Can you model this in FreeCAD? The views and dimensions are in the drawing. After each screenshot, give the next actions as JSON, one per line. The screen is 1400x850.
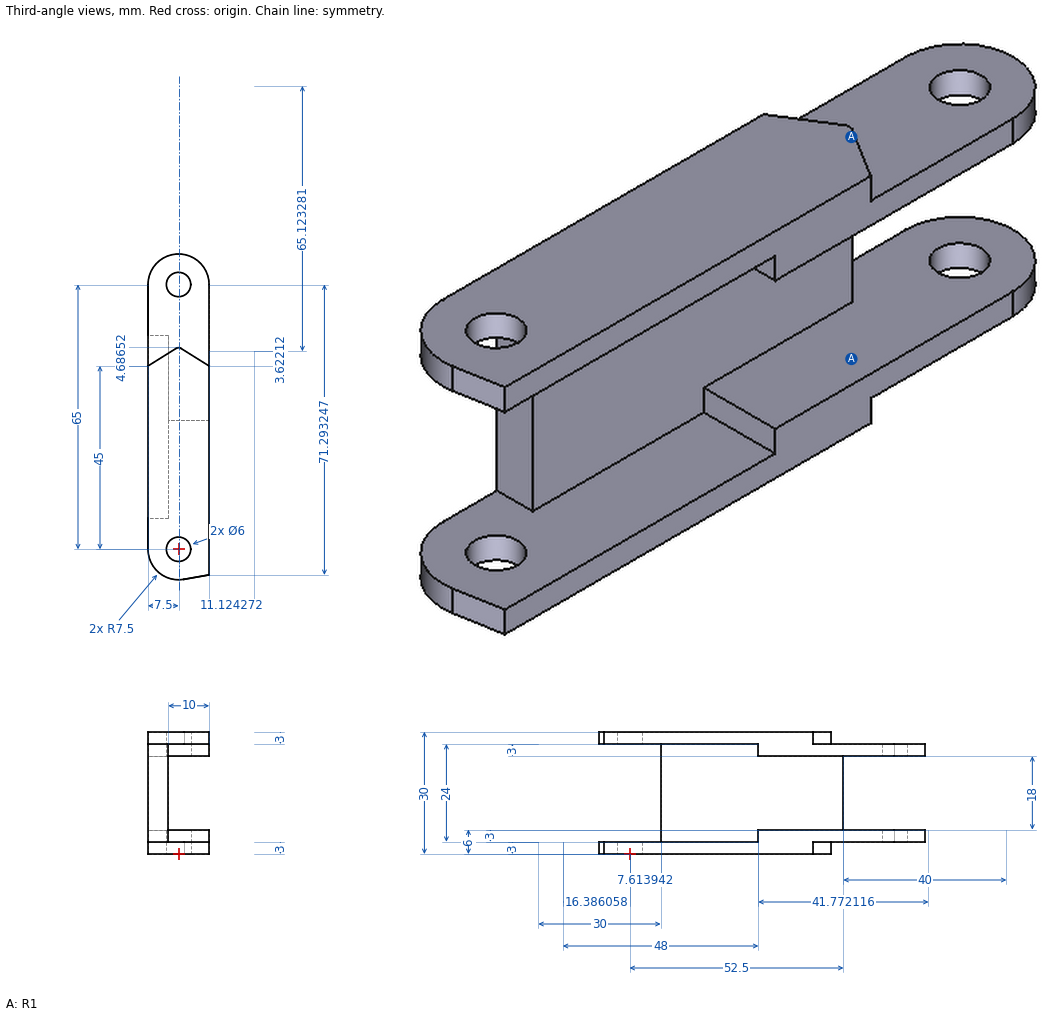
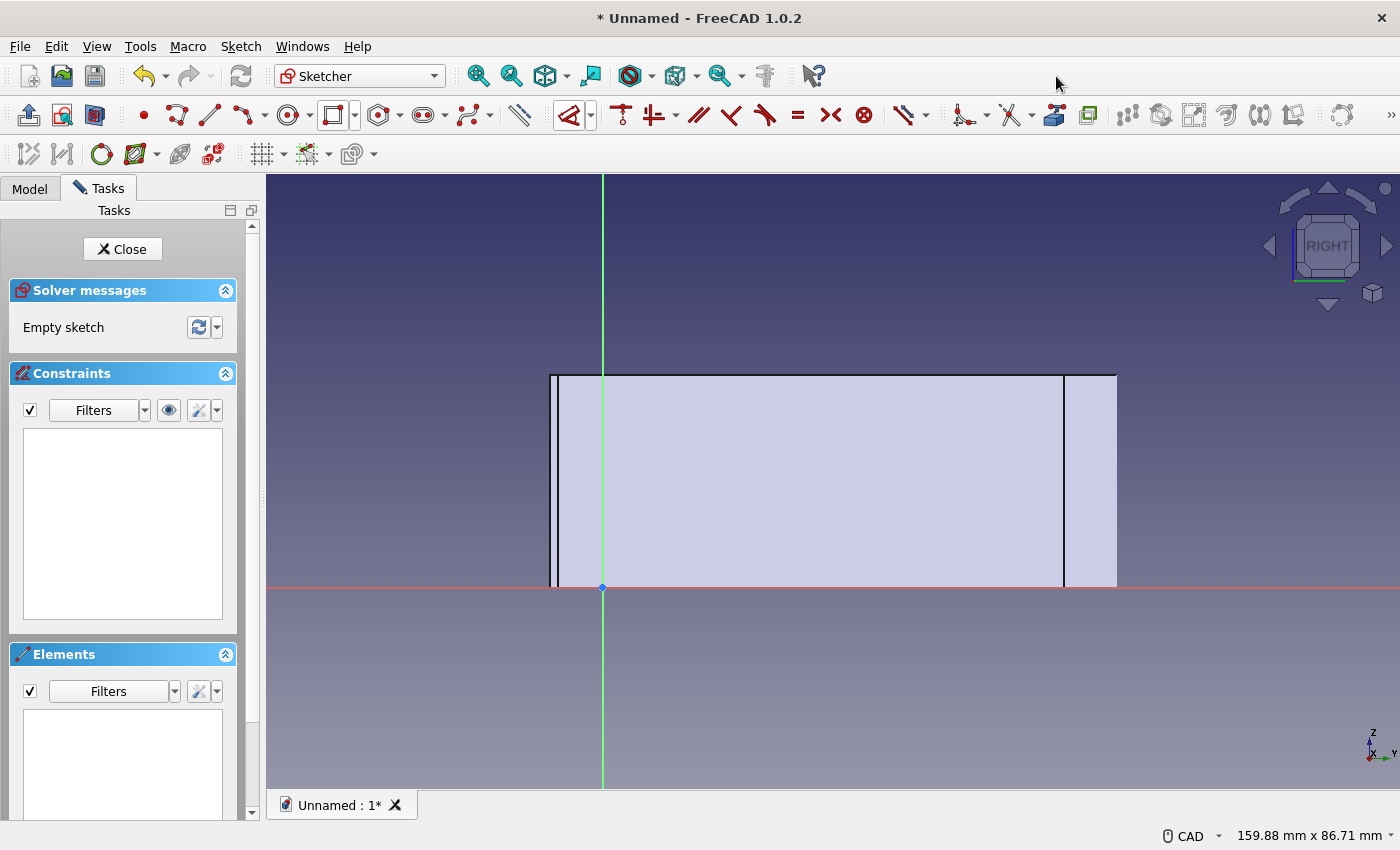
{"action": "scroll", "coordinate": [373, 433], "scroll_direction": "down", "scroll_amount": 1}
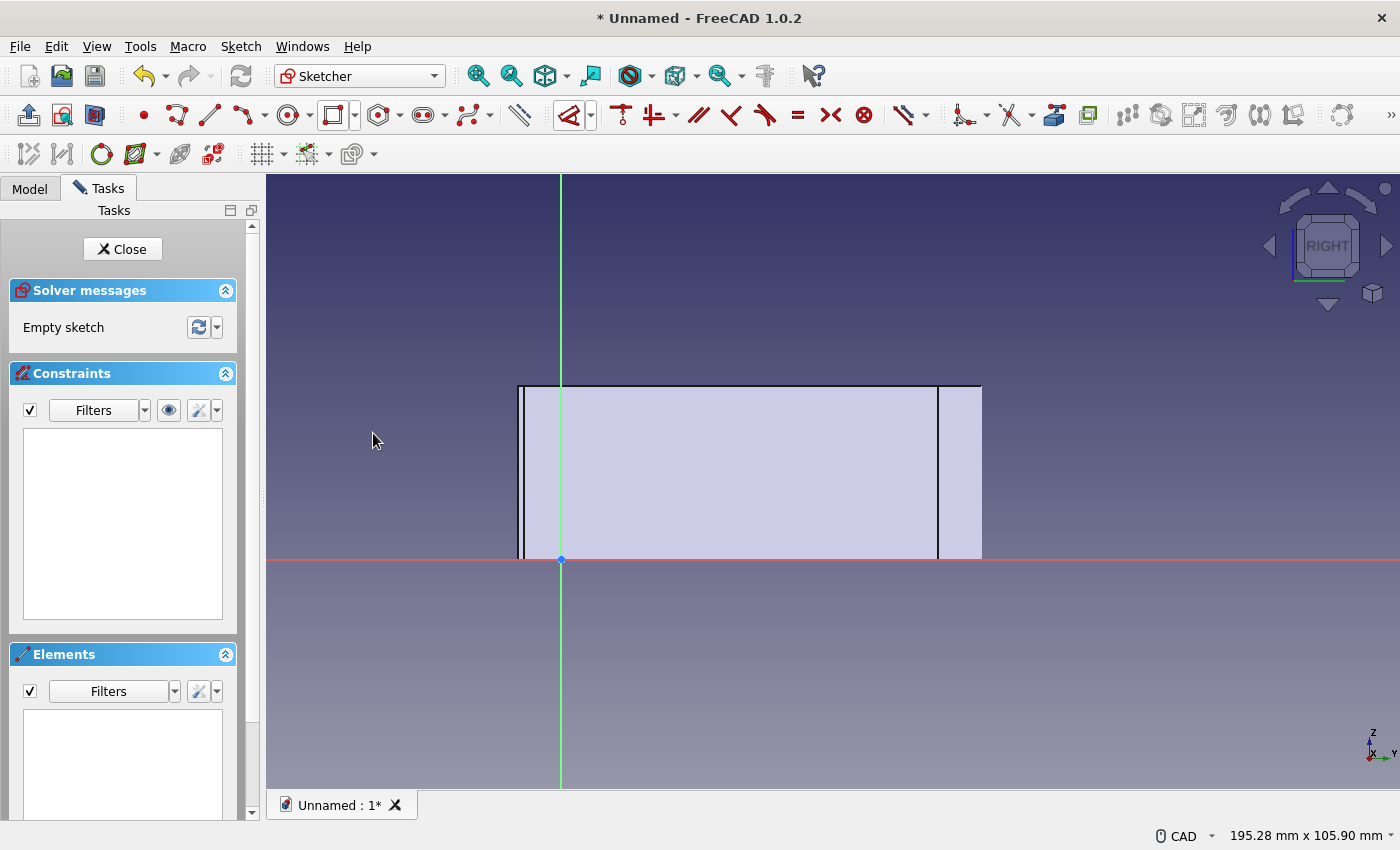
{"action": "key", "text": "g r"}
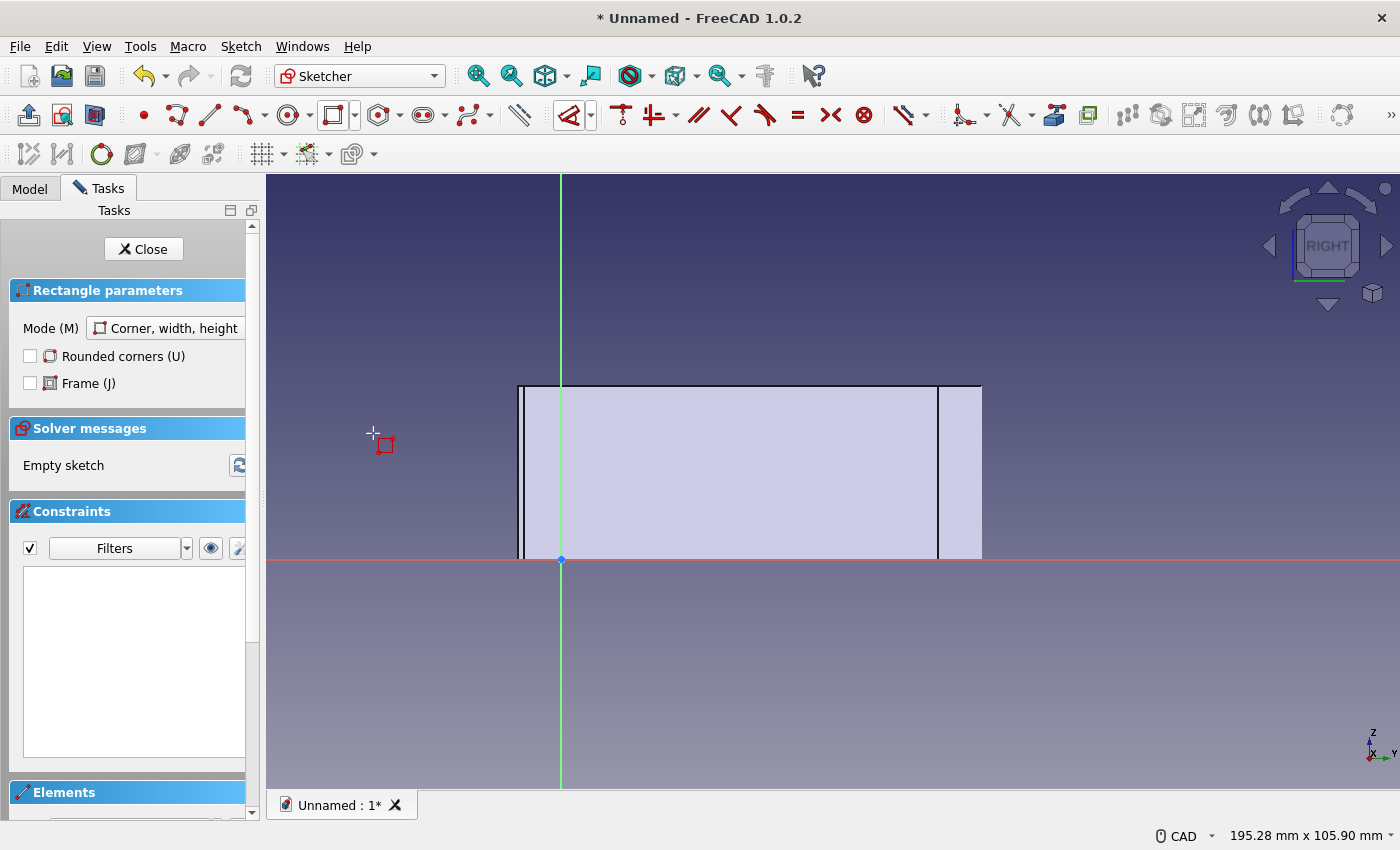
{"action": "left_click", "coordinate": [431, 403]}
{"action": "left_click", "coordinate": [605, 542]}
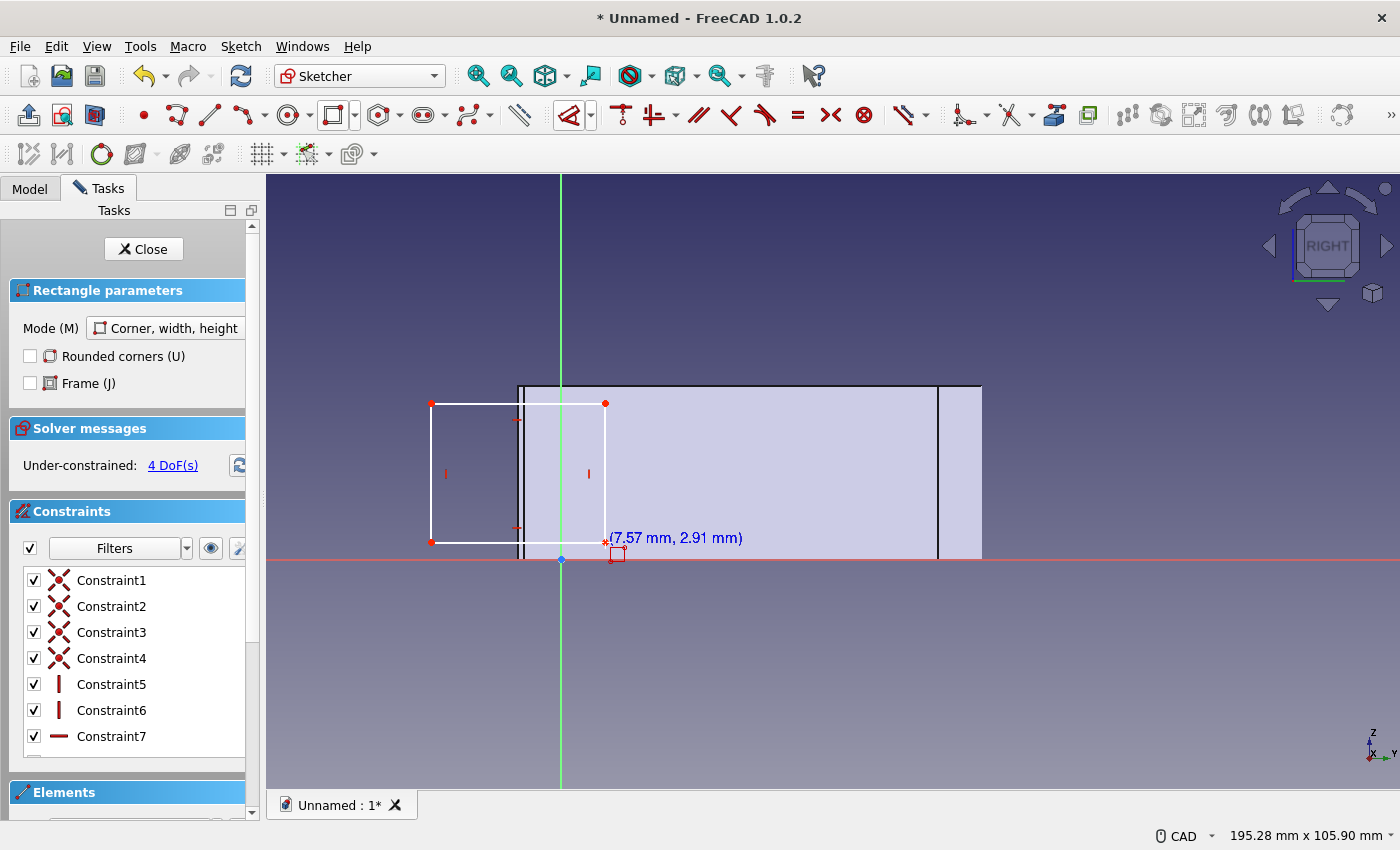
{"action": "left_click", "coordinate": [866, 421]}
{"action": "left_click", "coordinate": [1098, 525]}
{"action": "key", "text": "Escape"}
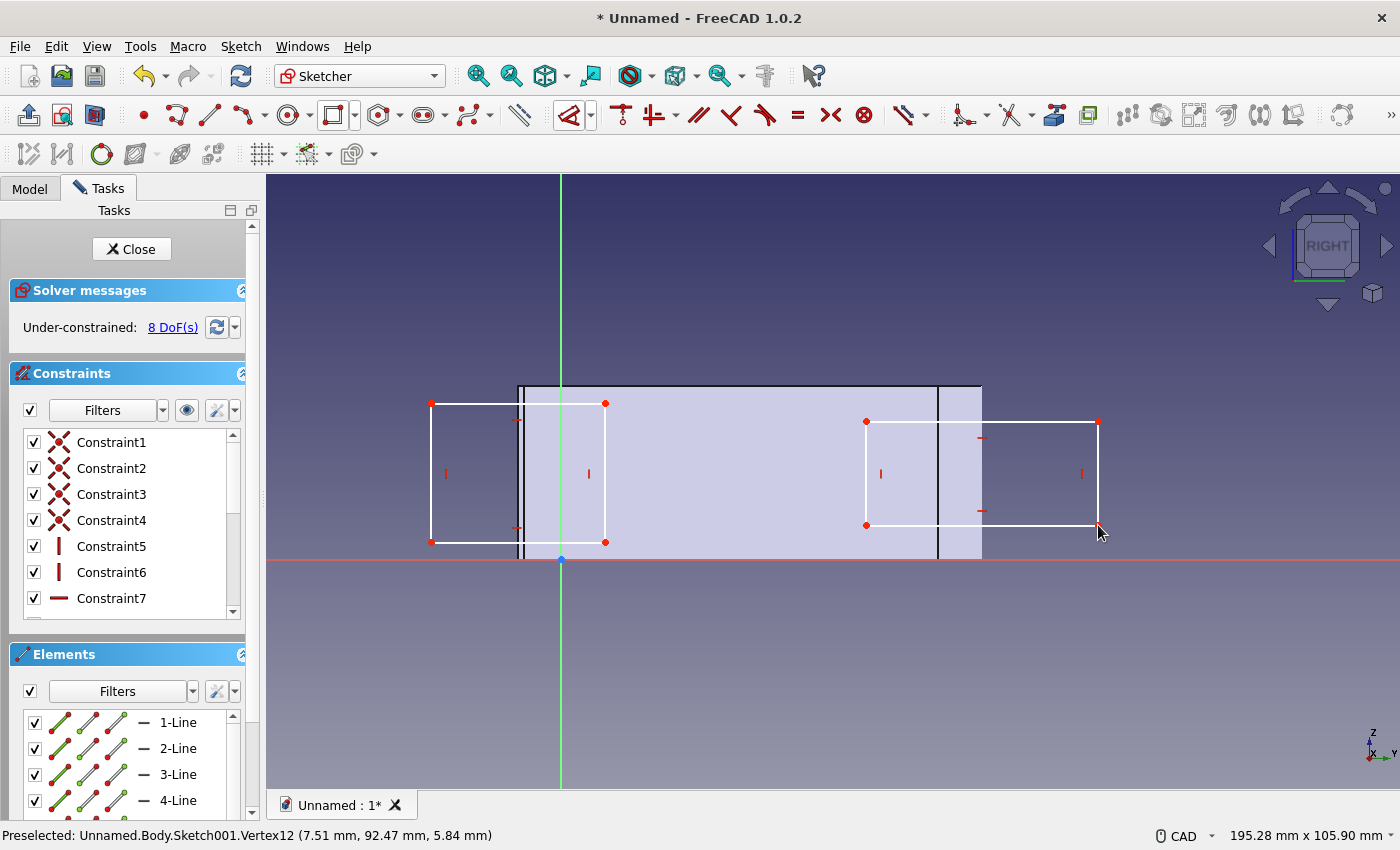
{"action": "left_click", "coordinate": [431, 446]}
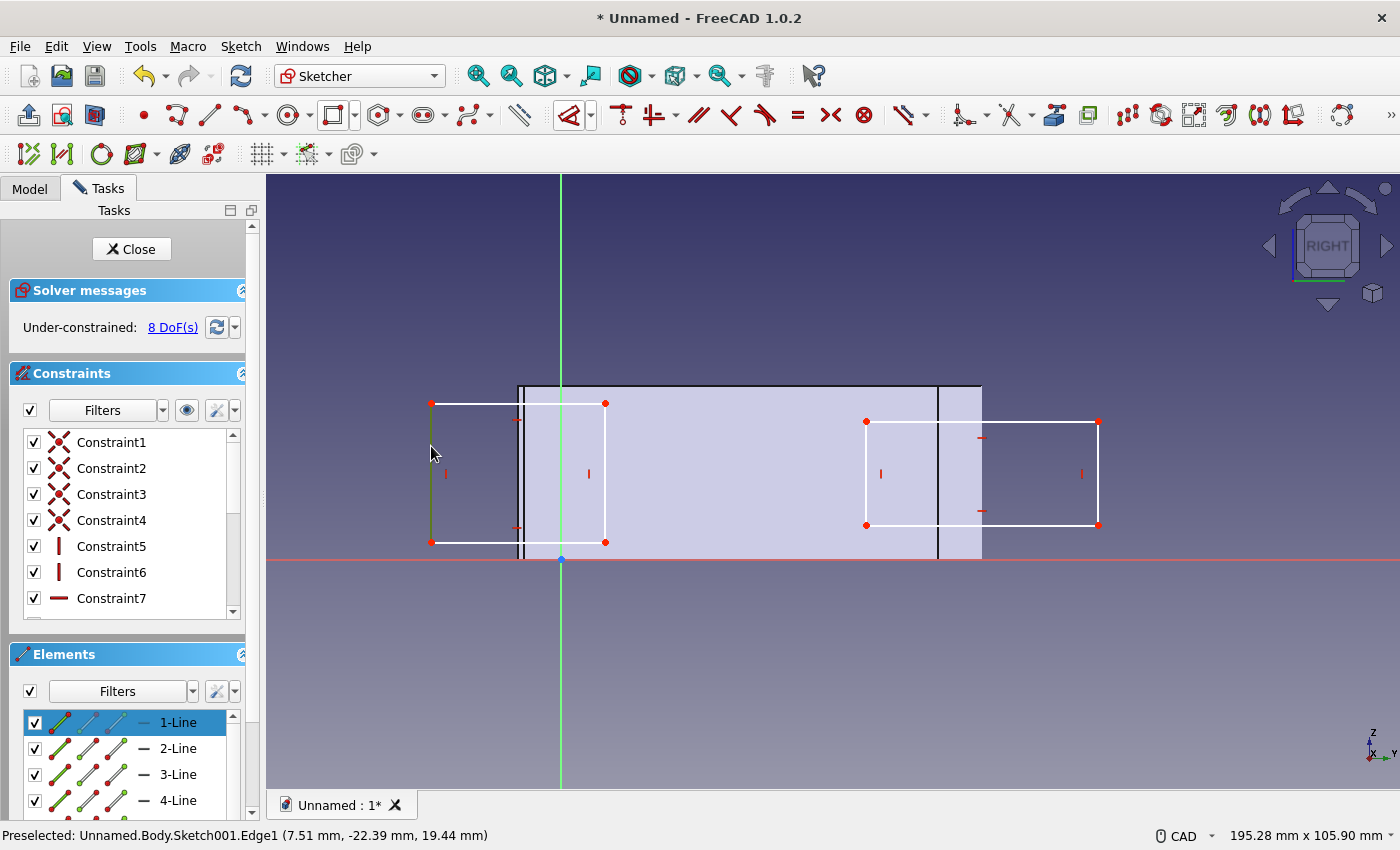
{"action": "left_click", "coordinate": [590, 116]}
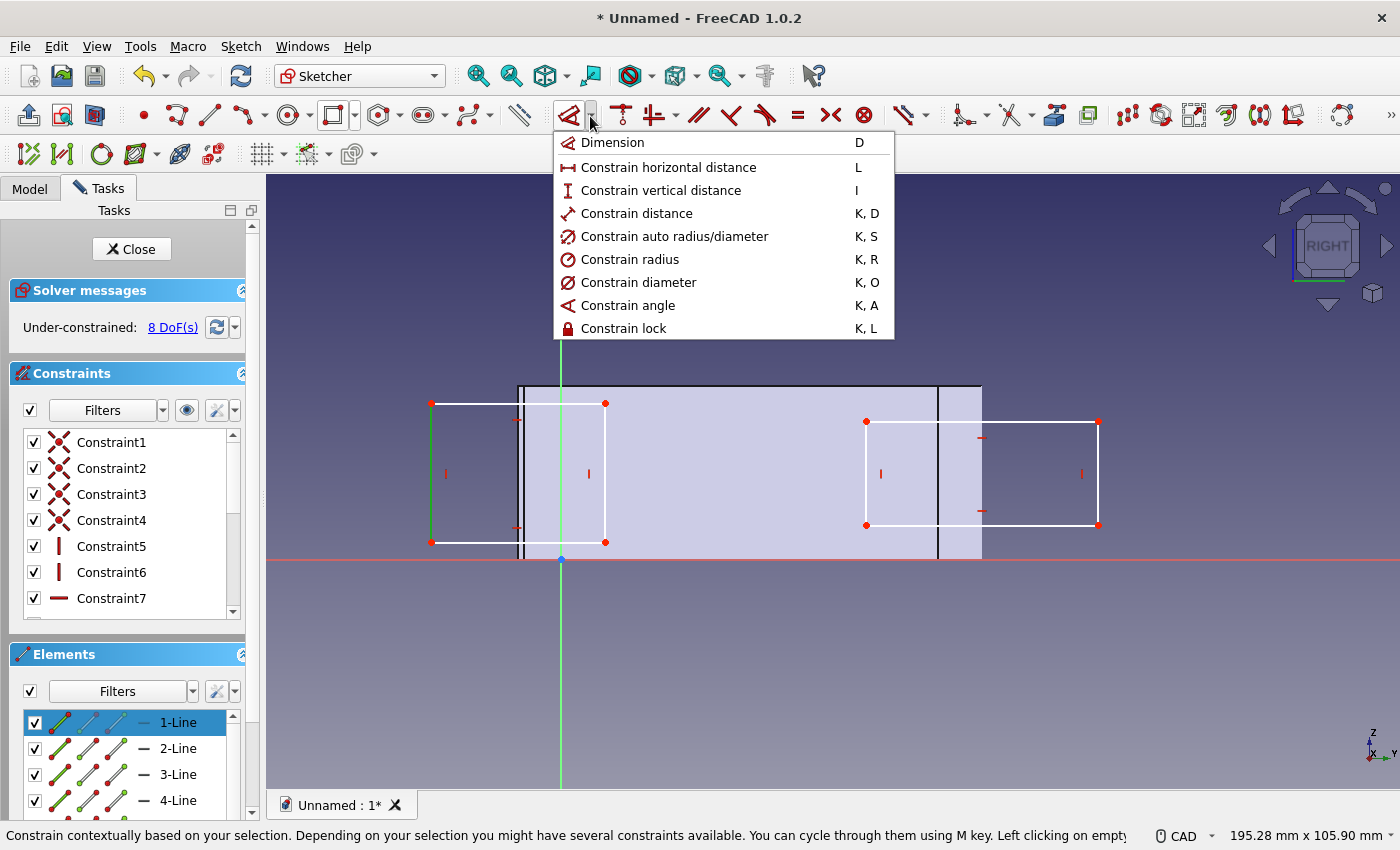
{"action": "left_click", "coordinate": [724, 190]}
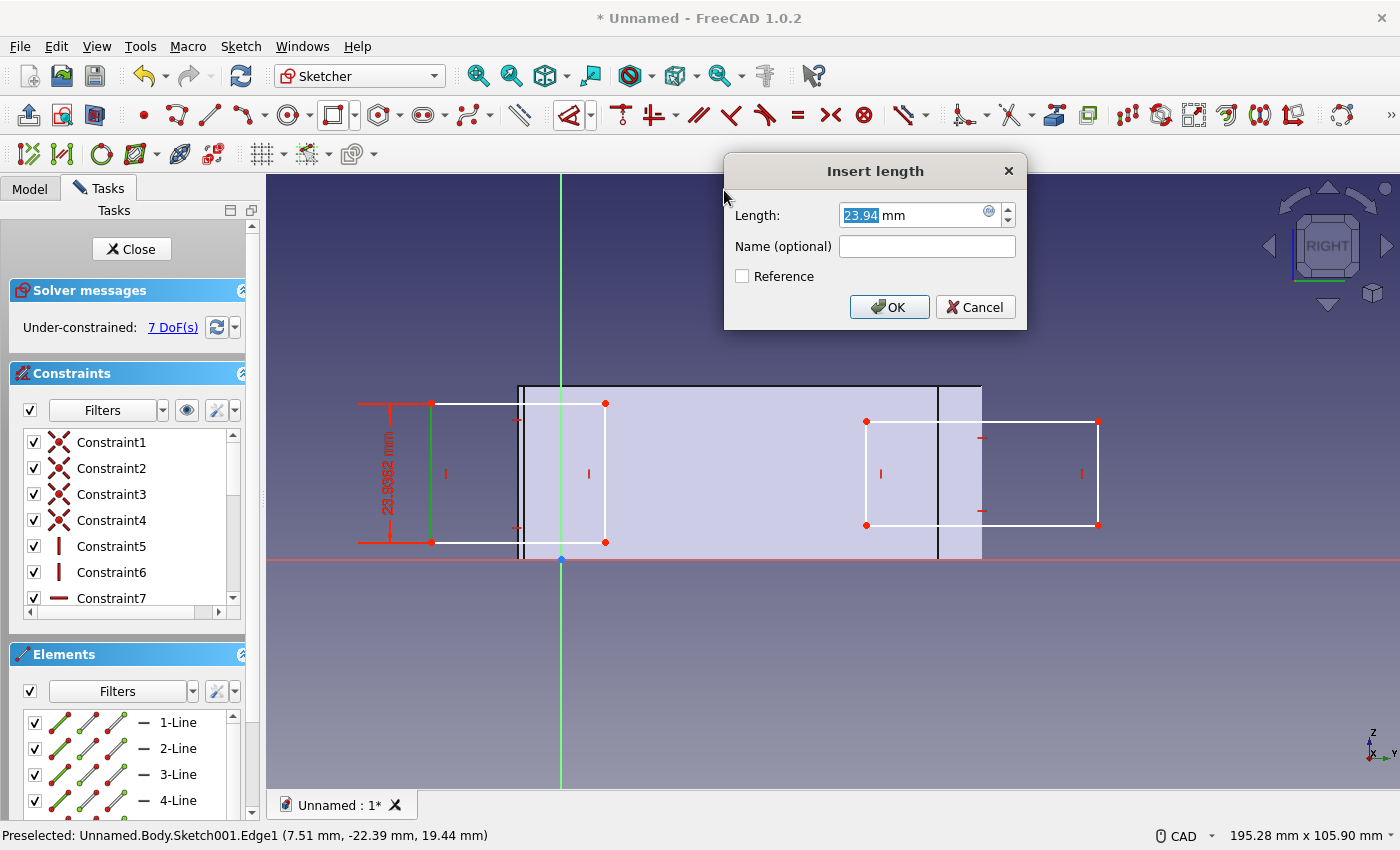
{"action": "type", "text": "24"}
{"action": "key", "text": "Return"}